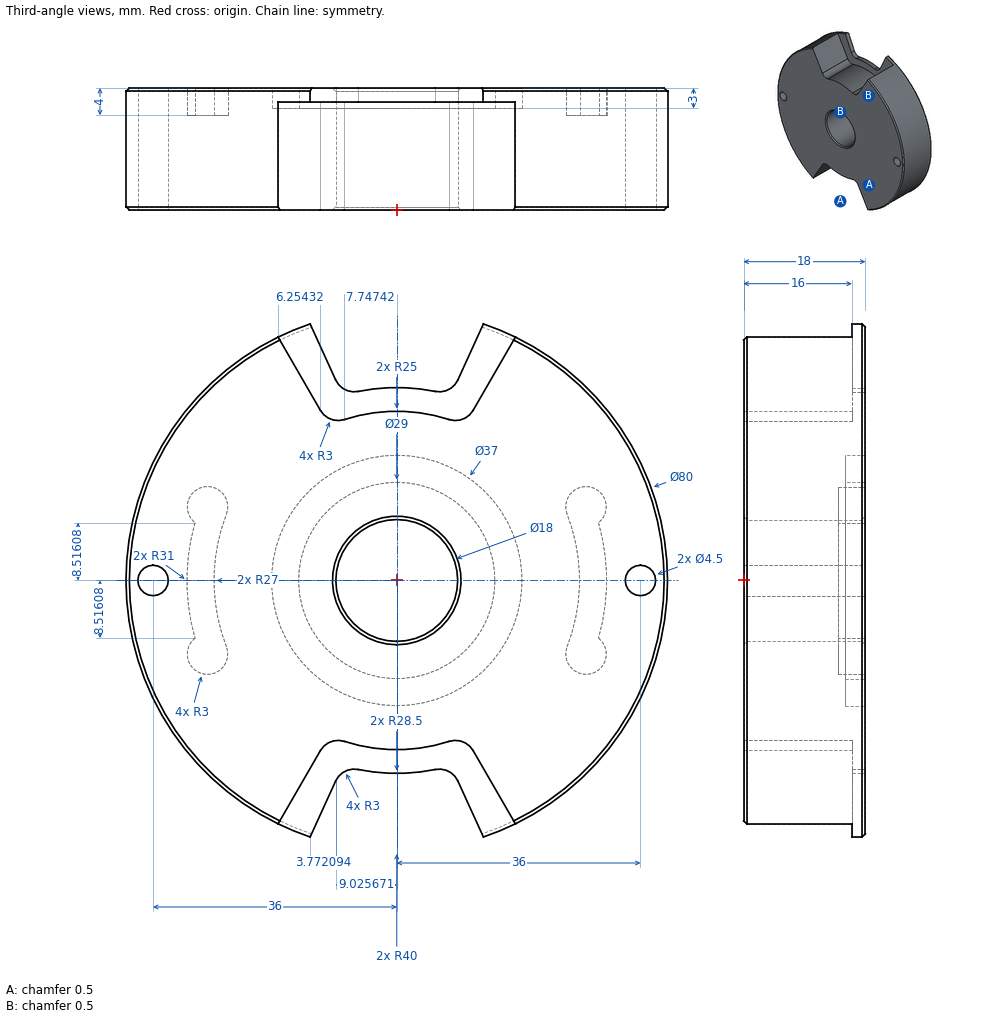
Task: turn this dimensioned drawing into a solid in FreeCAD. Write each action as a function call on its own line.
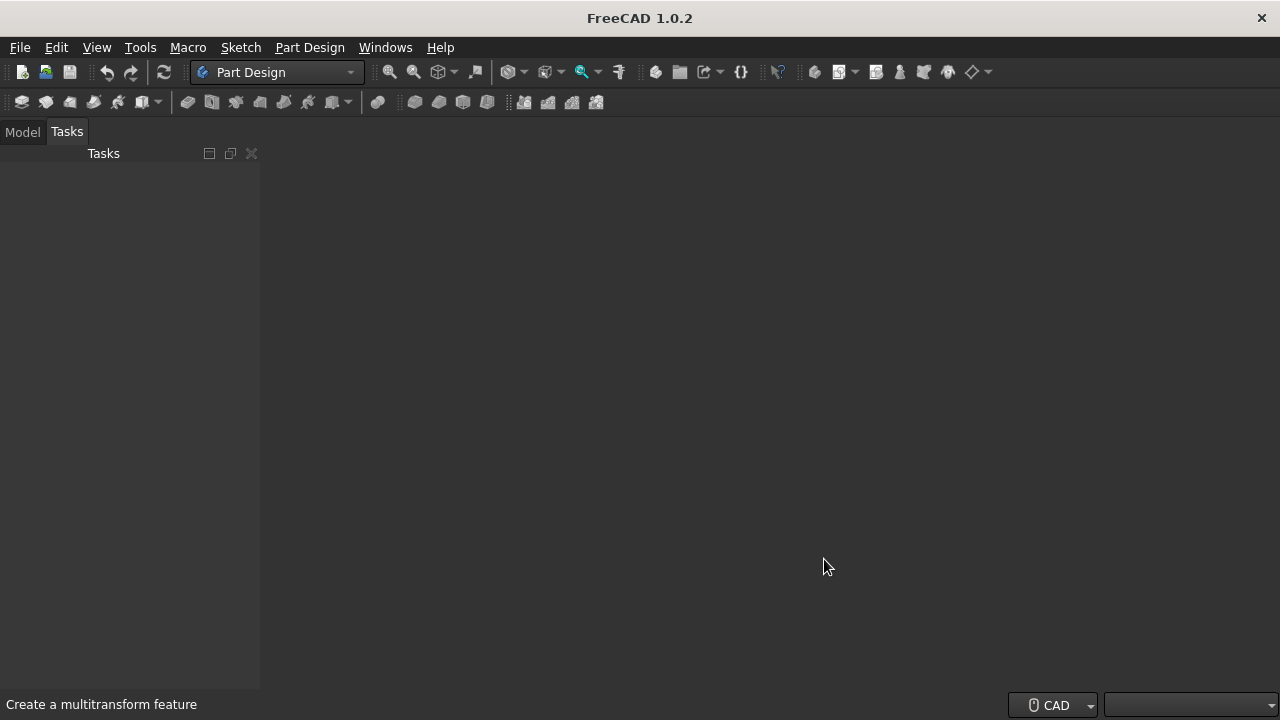
click(22, 72)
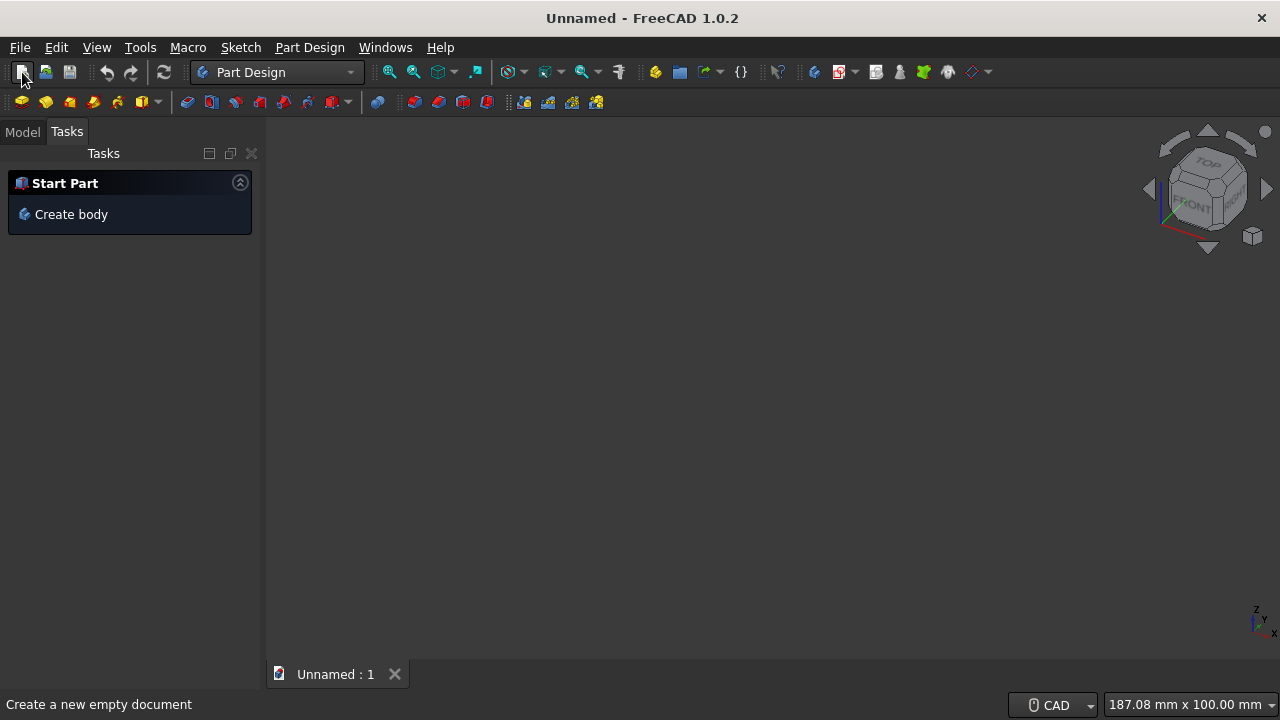
click(840, 72)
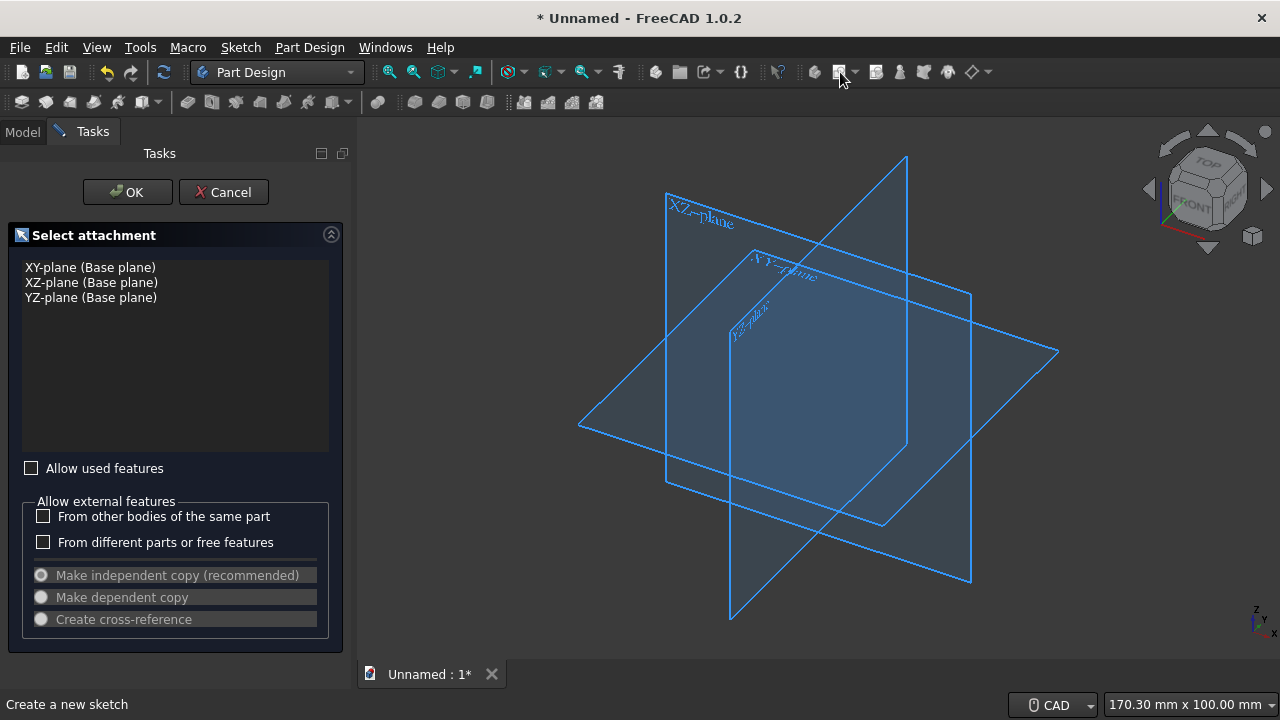
click(82, 282)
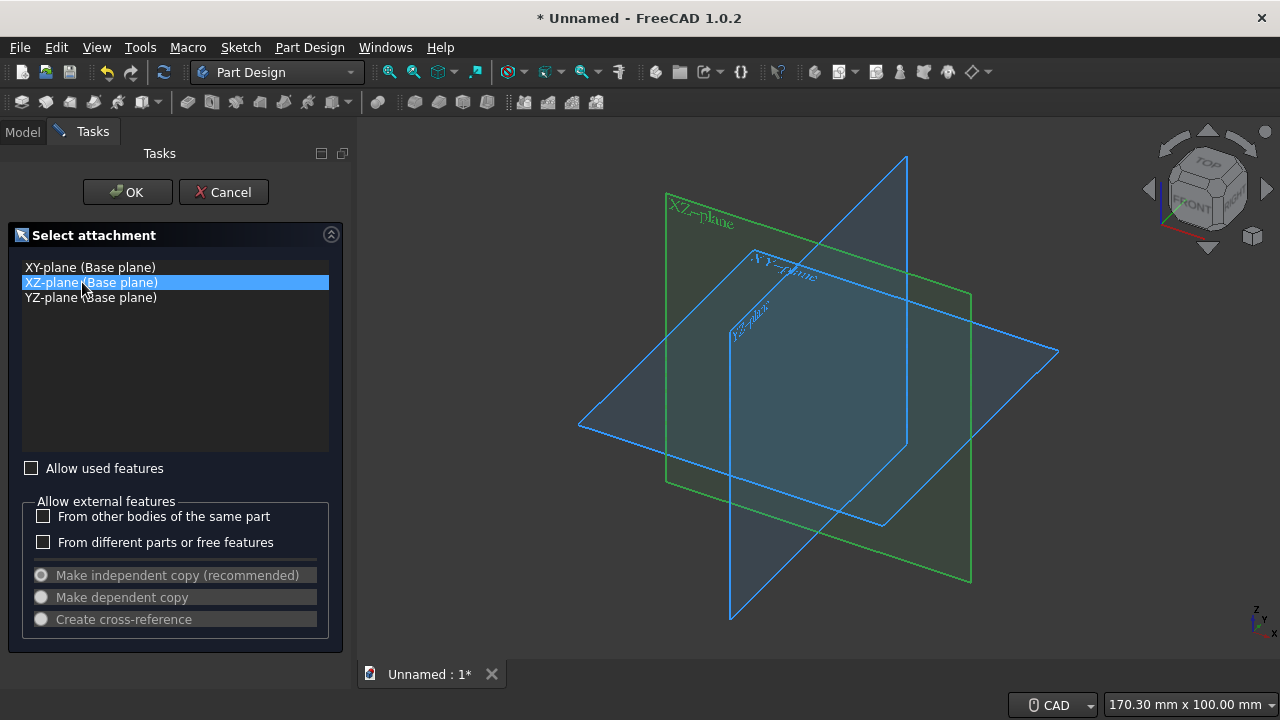
click(128, 192)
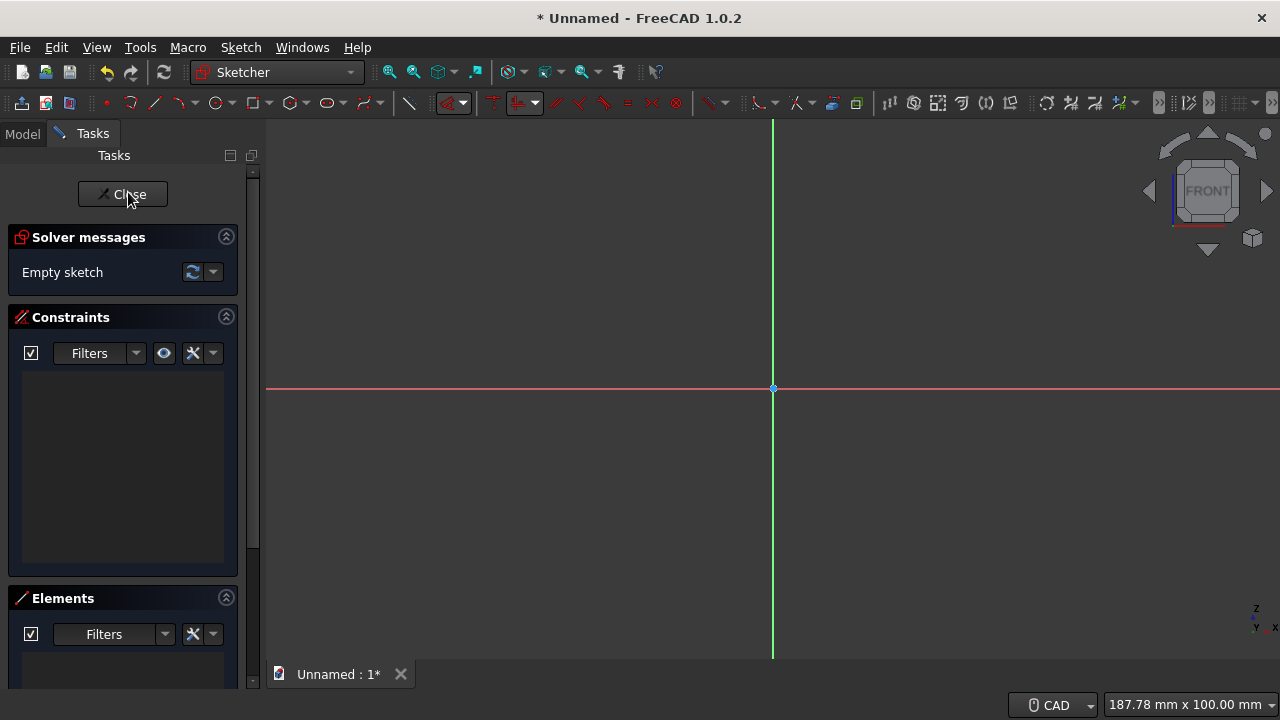
click(216, 104)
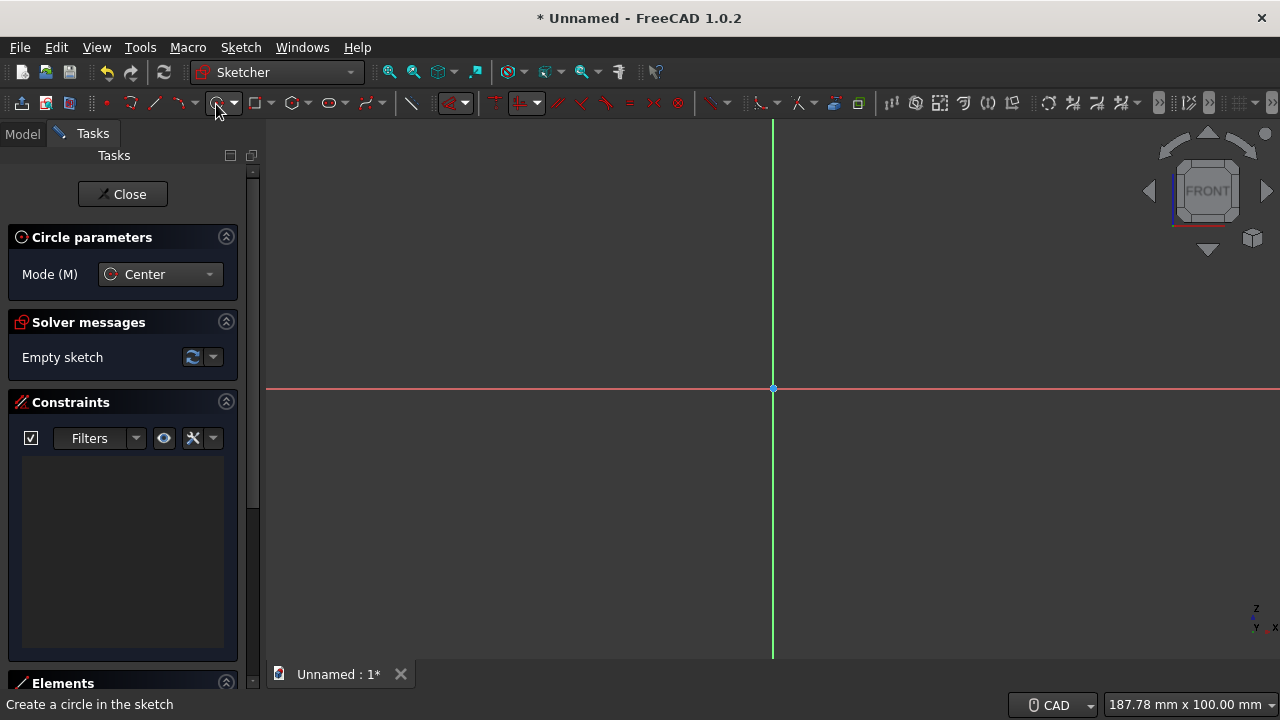
click(773, 389)
click(926, 236)
key(Escape)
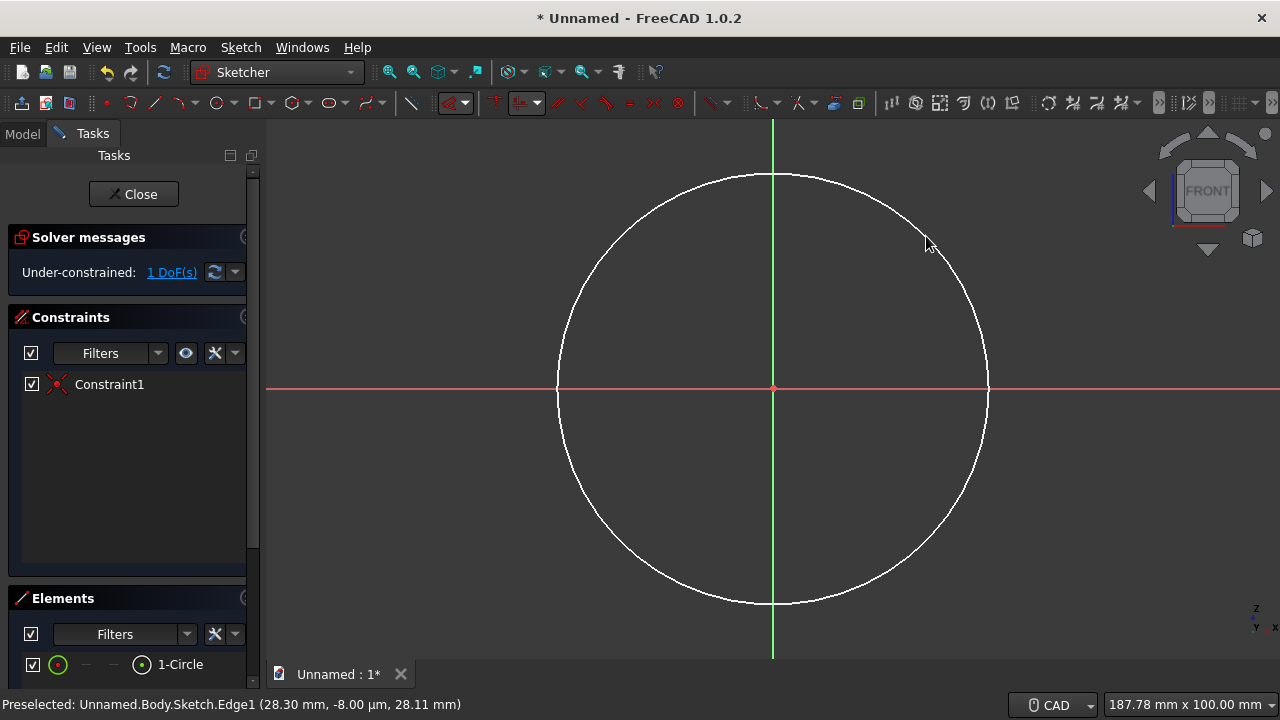
click(450, 104)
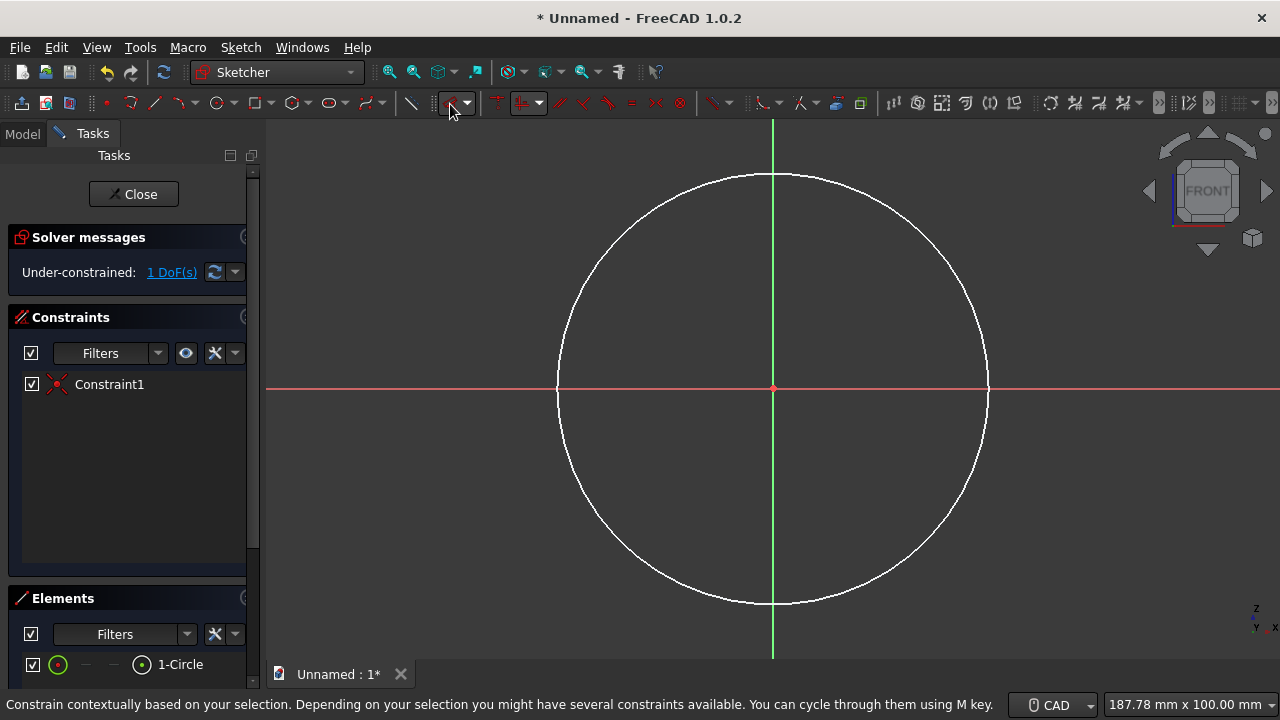
click(925, 236)
click(948, 213)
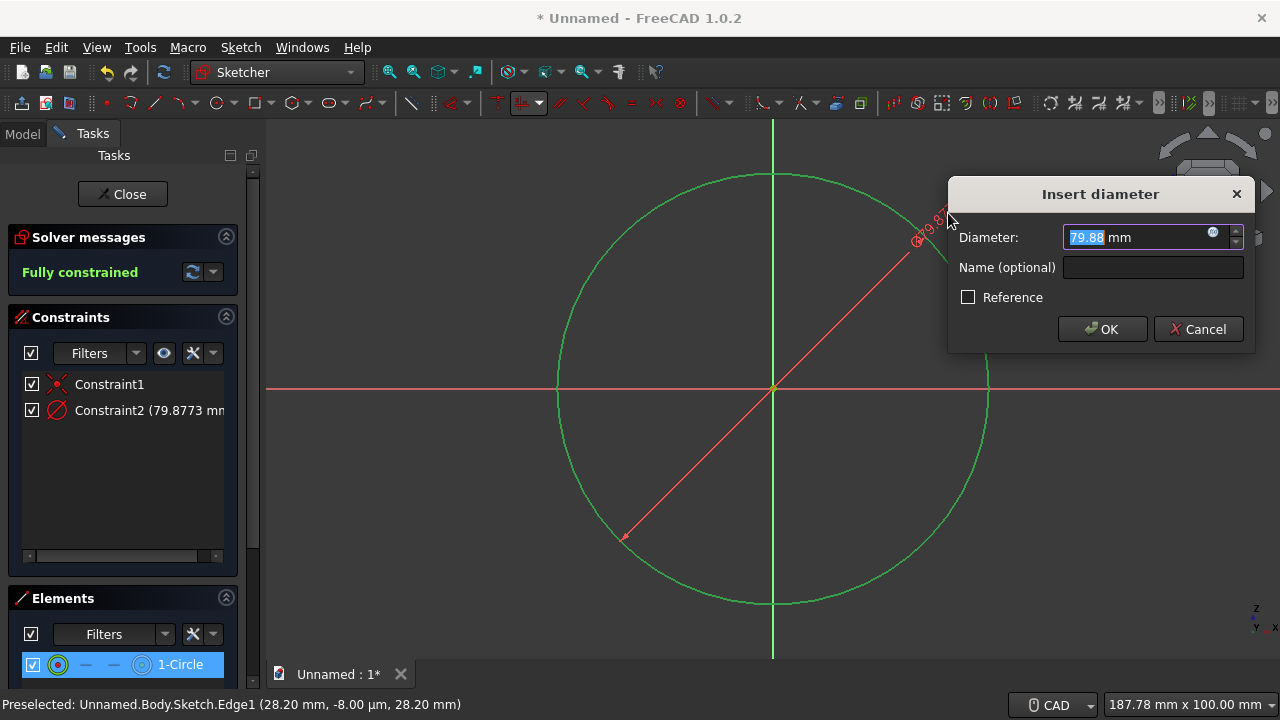
text(80)
key(Return)
key(Escape)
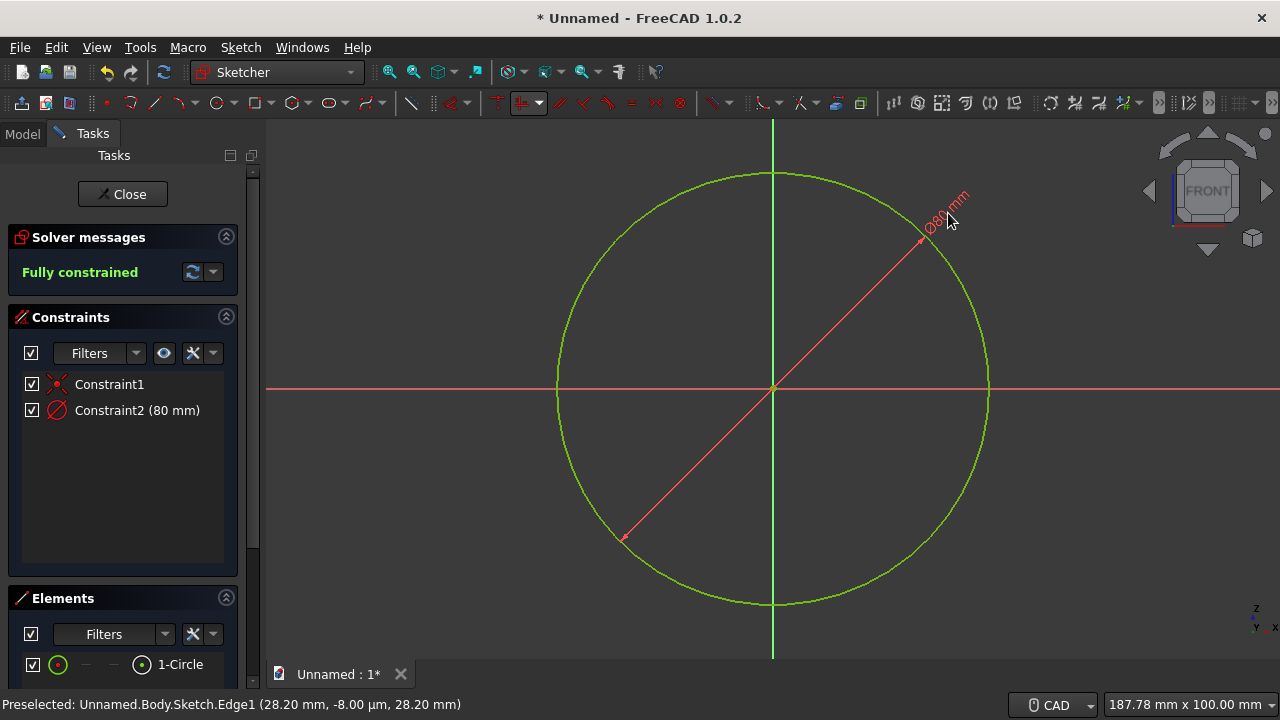
click(123, 194)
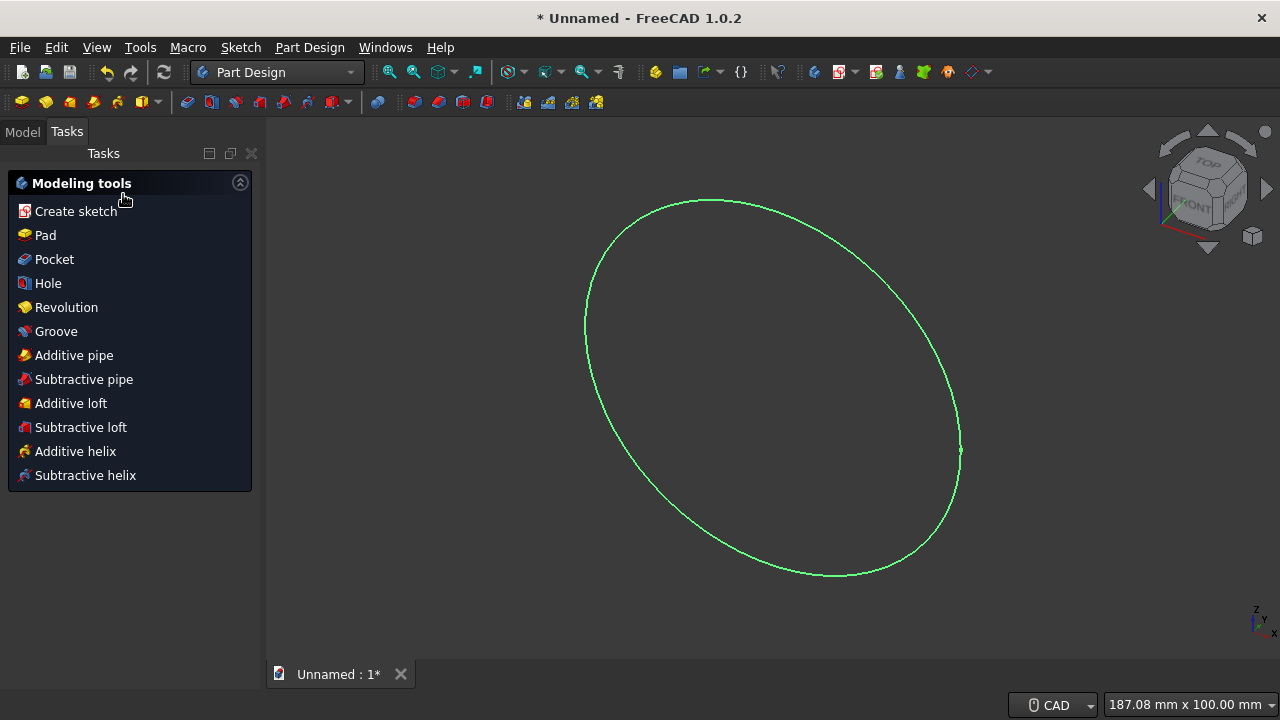
click(22, 102)